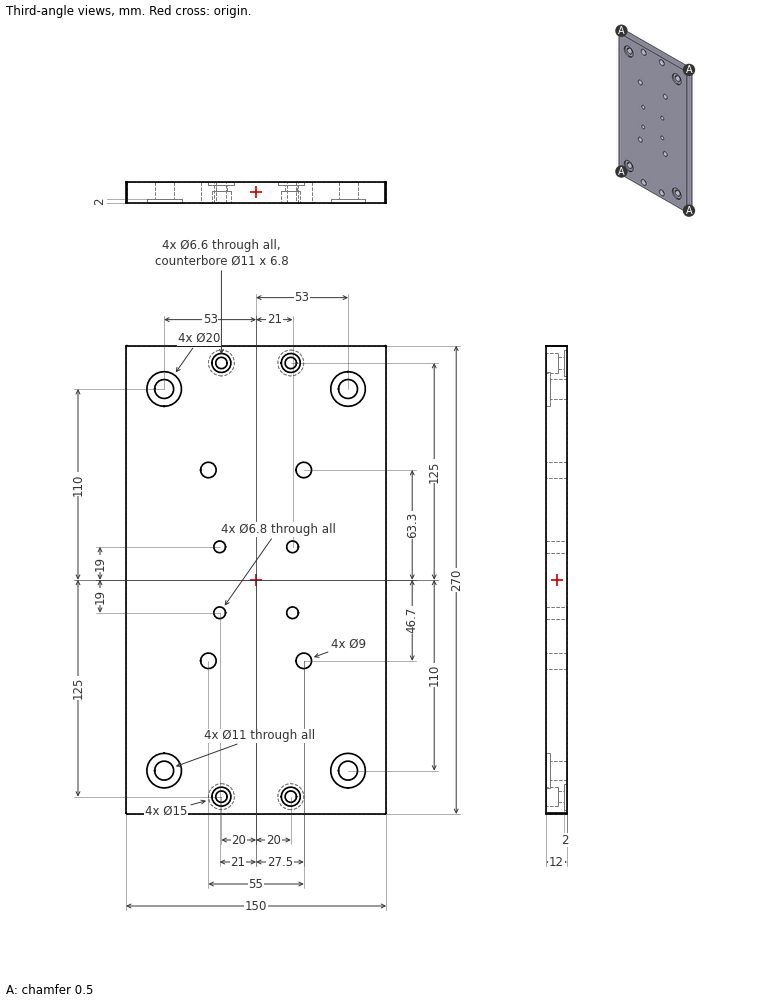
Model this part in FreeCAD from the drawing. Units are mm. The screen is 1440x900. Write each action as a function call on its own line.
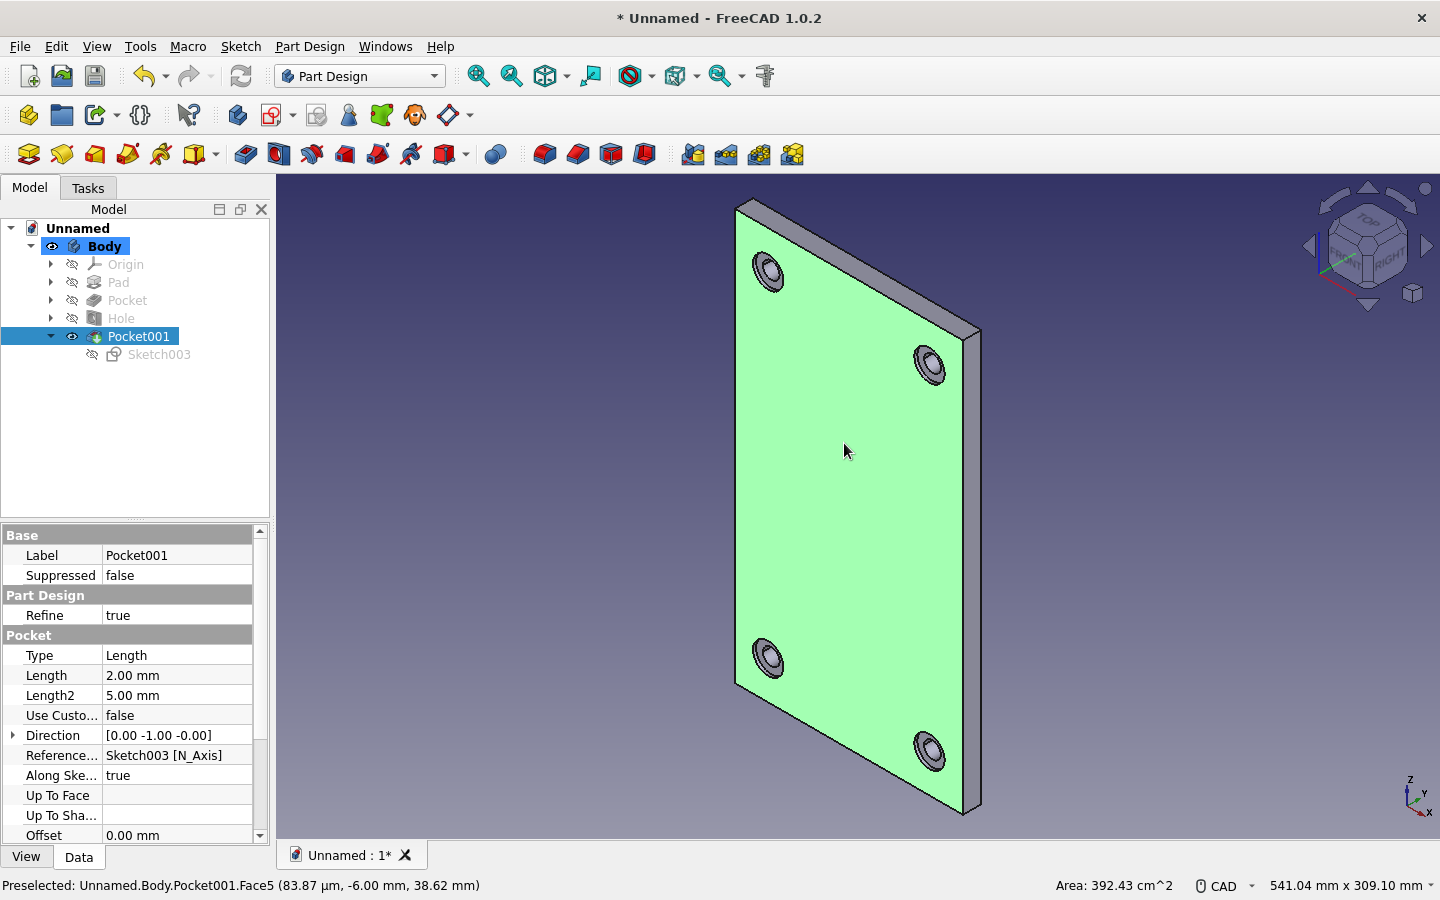
click(270, 116)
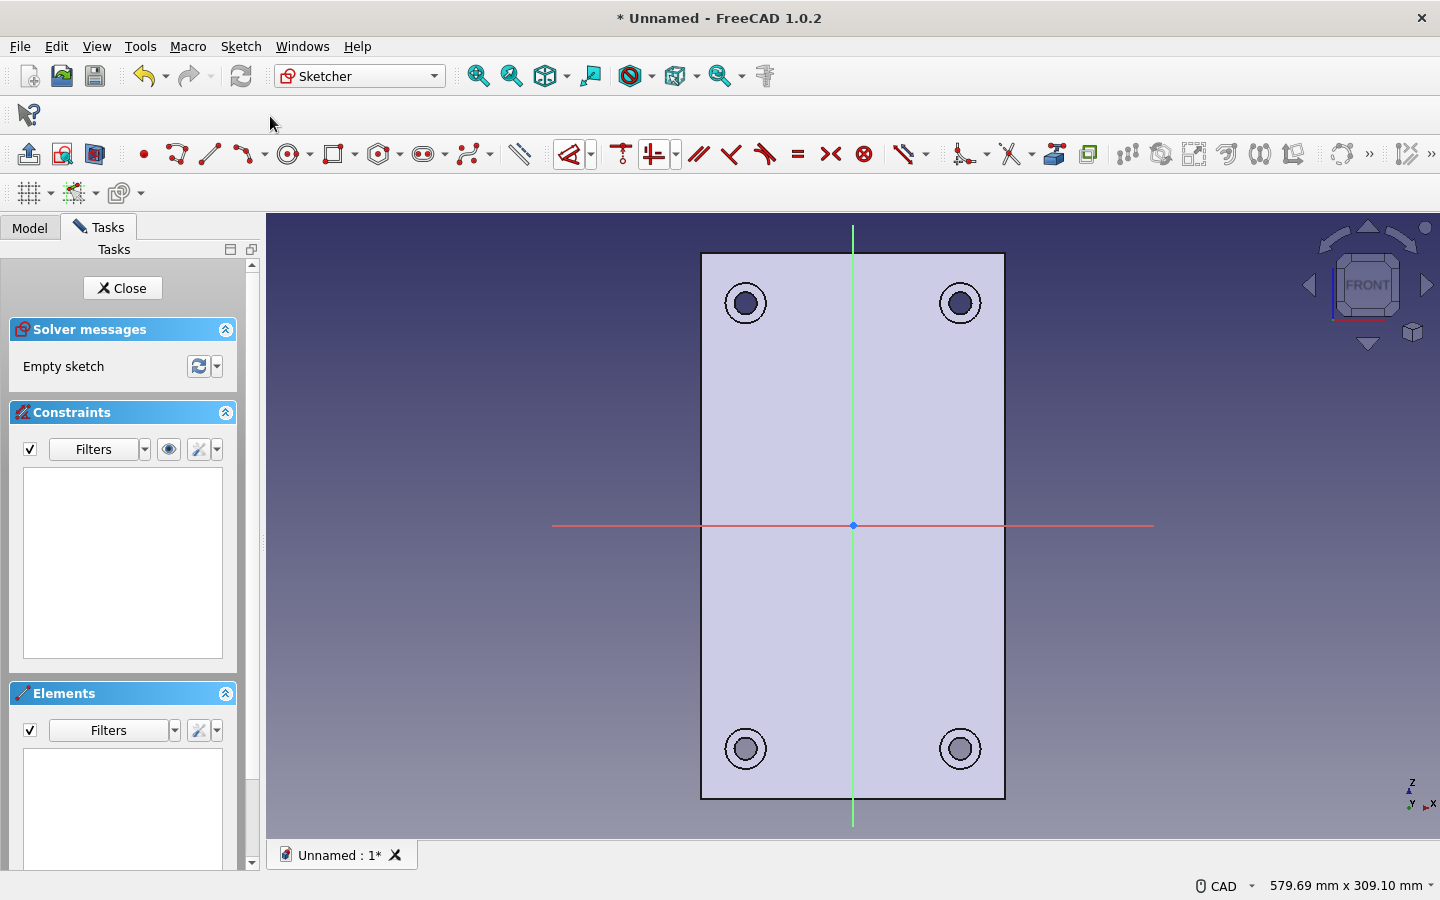
key(g)
key(c)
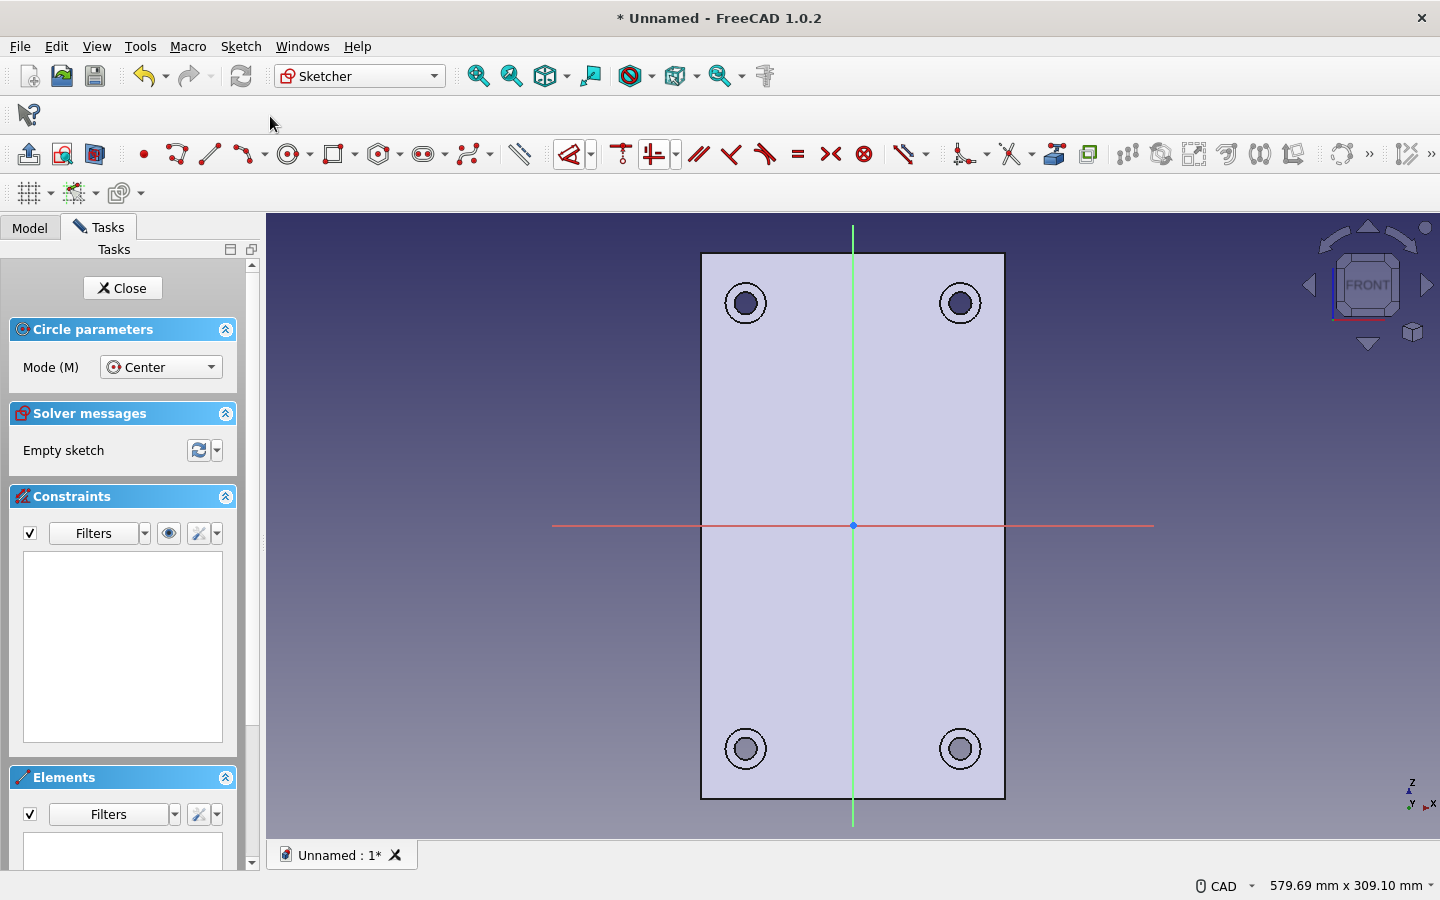
scroll(812, 273, up, 7)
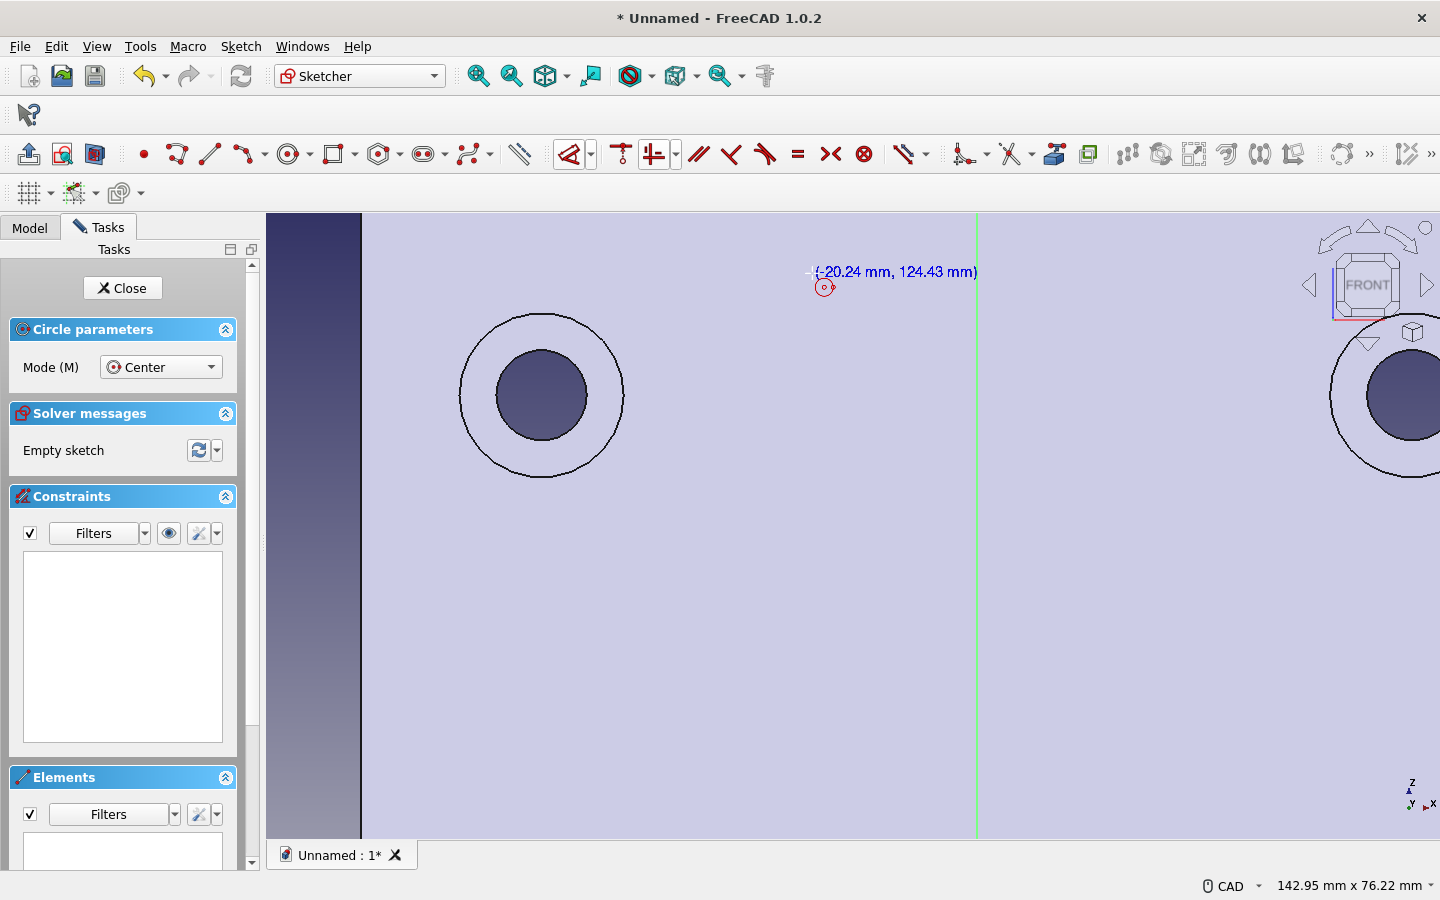
scroll(736, 331, down, 8)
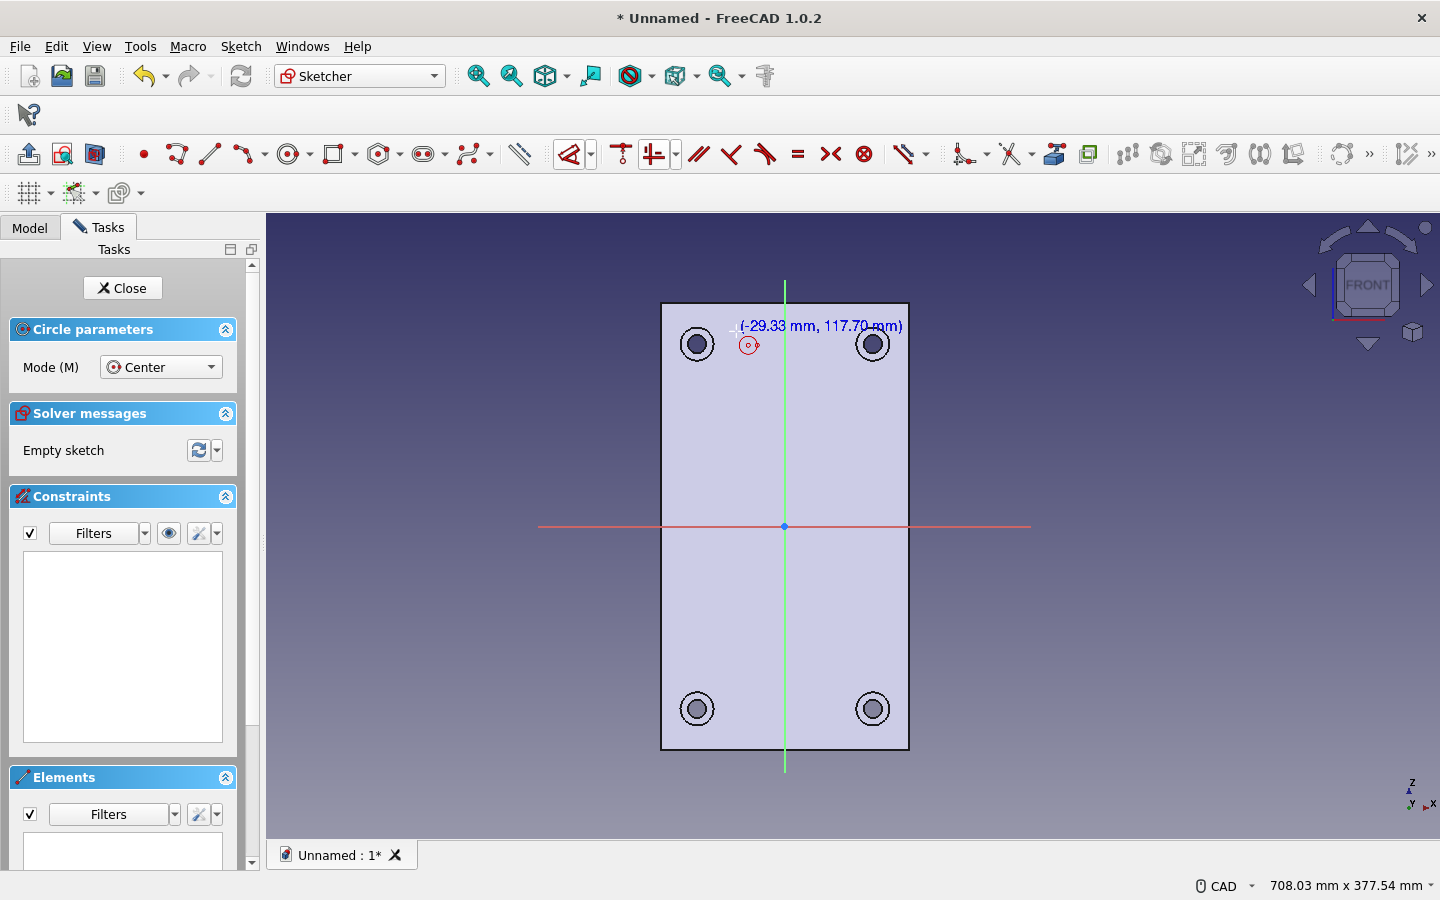
click(752, 319)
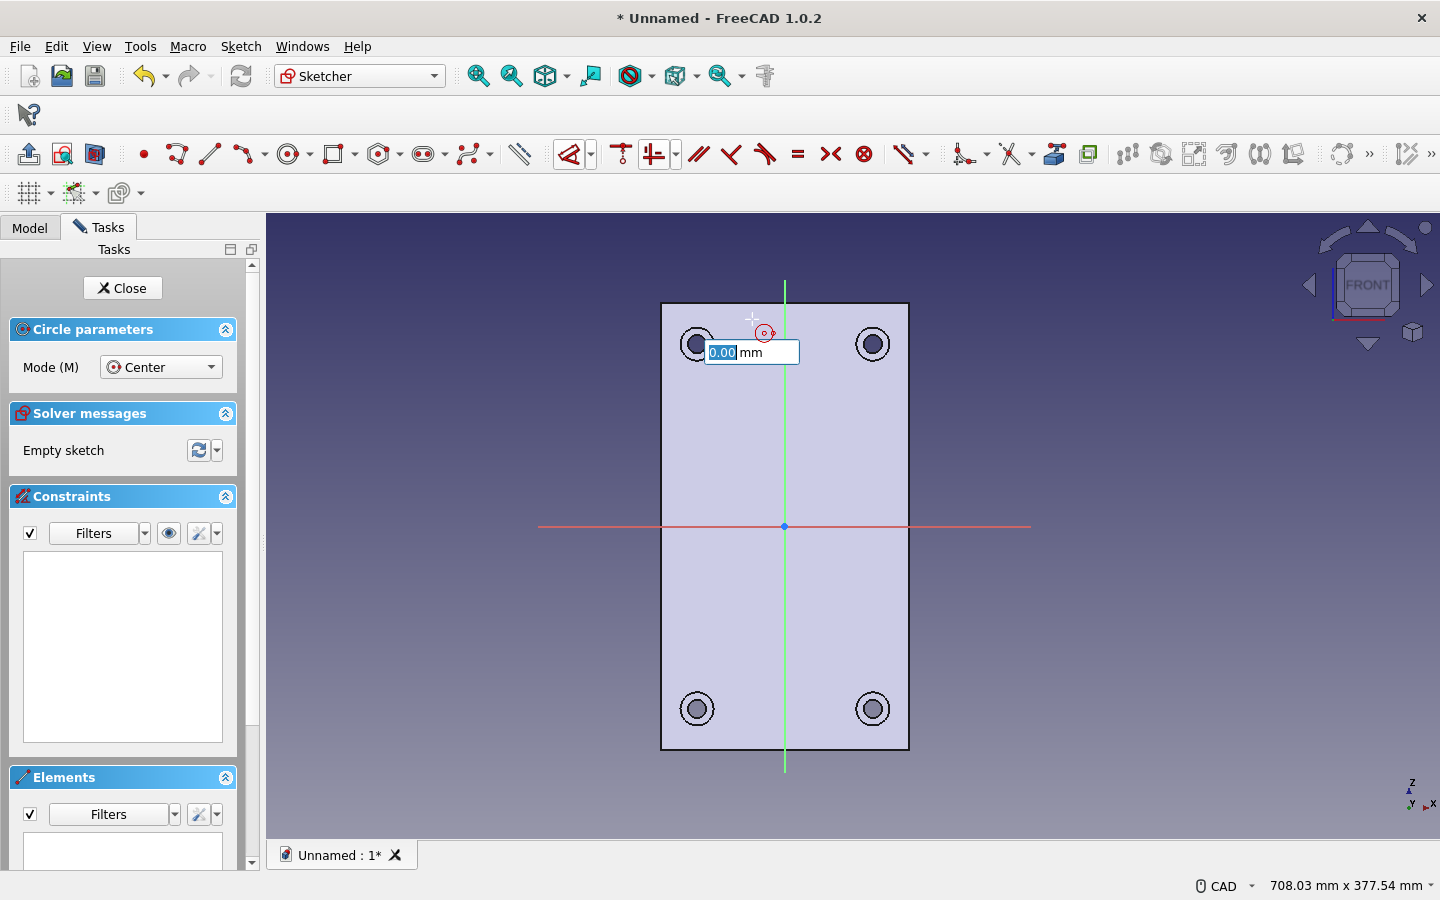
scroll(756, 315, up, 6)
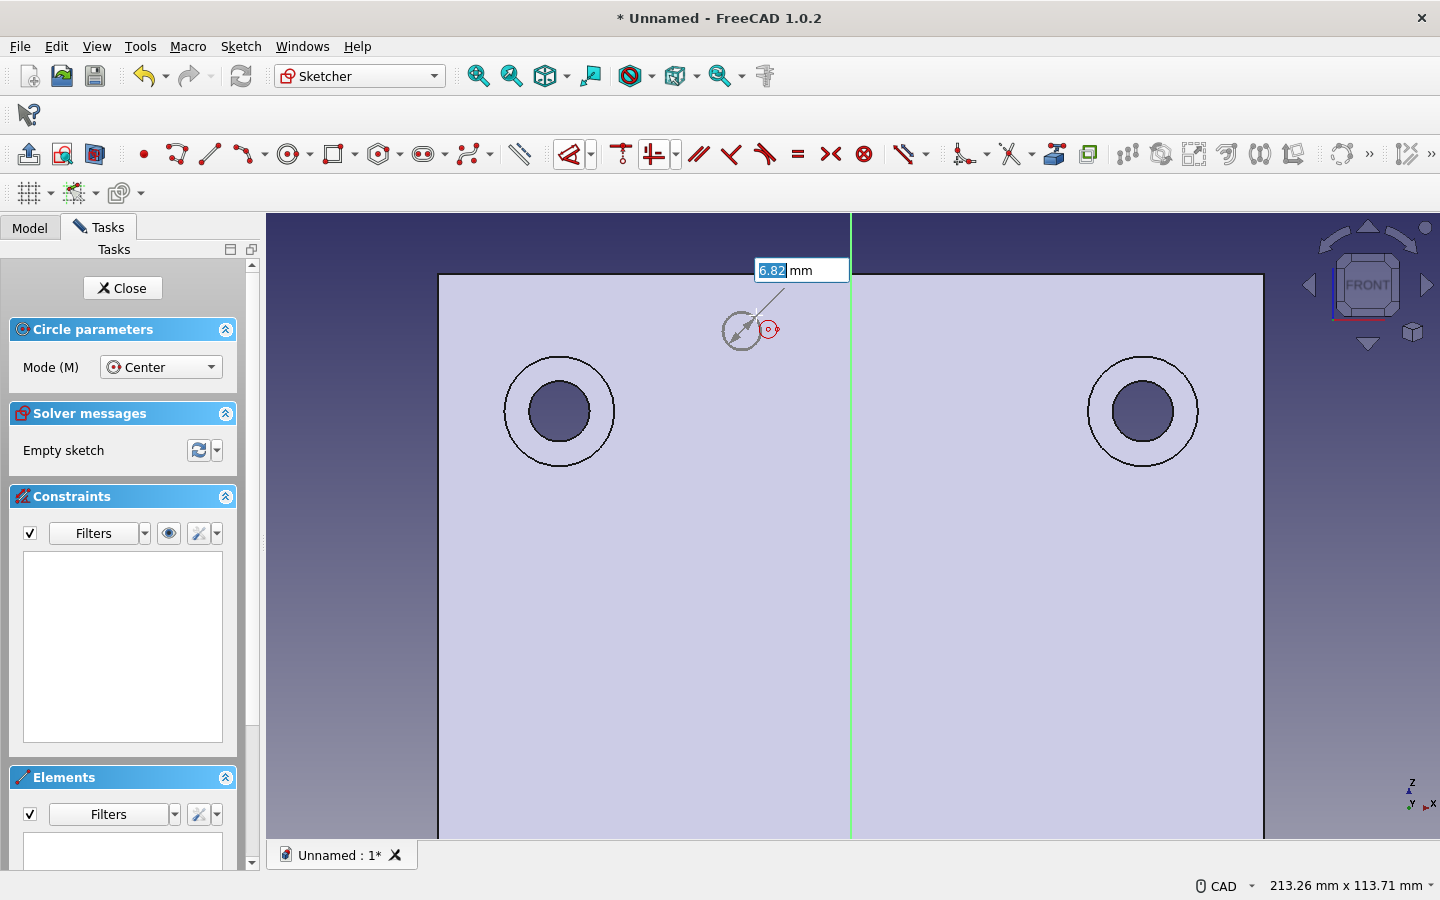
click(754, 316)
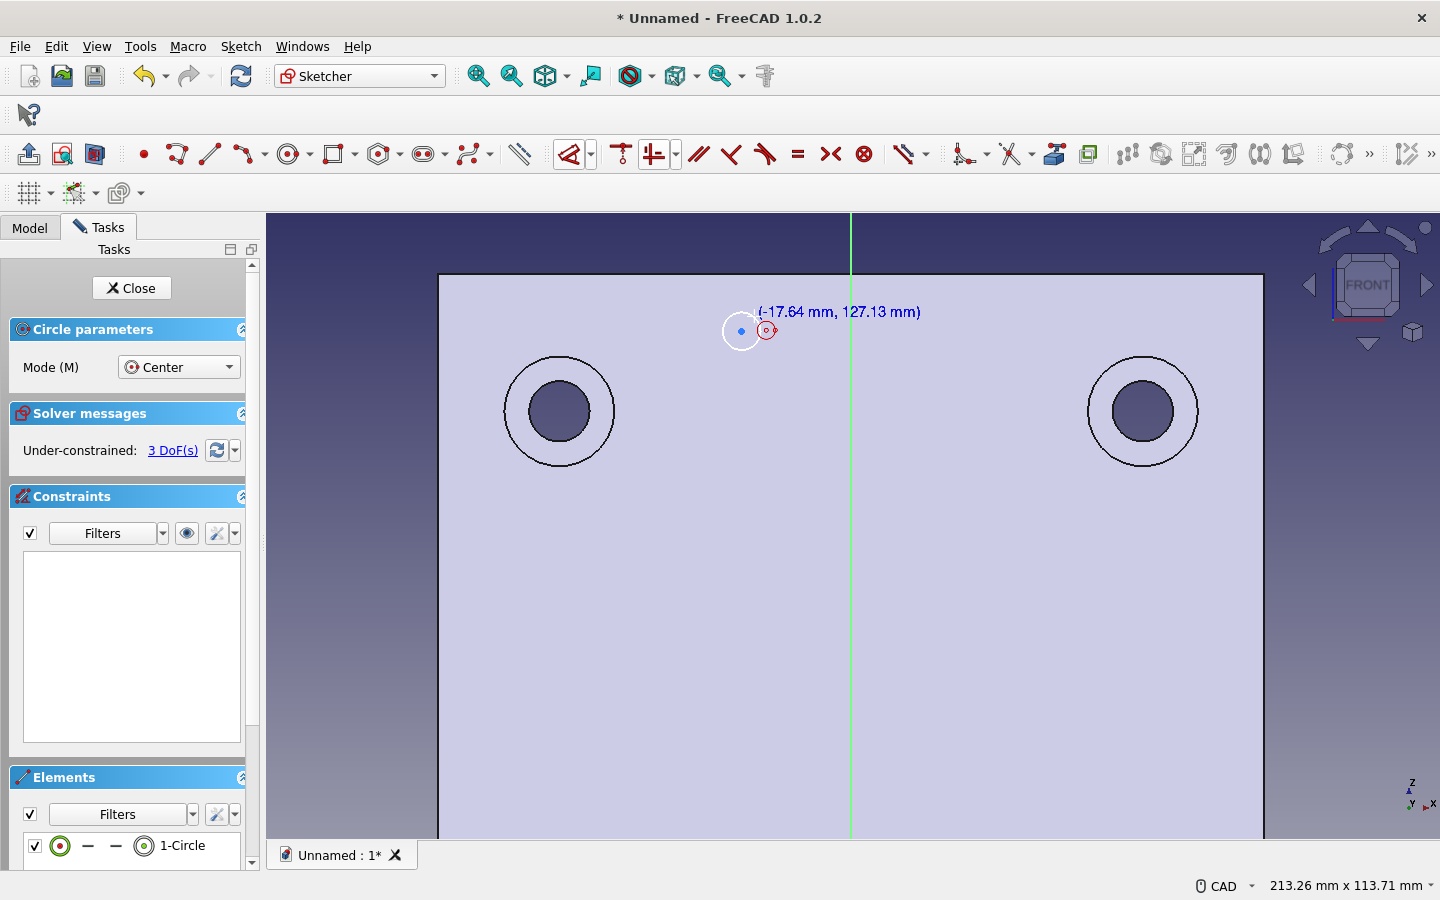
scroll(961, 329, up, 2)